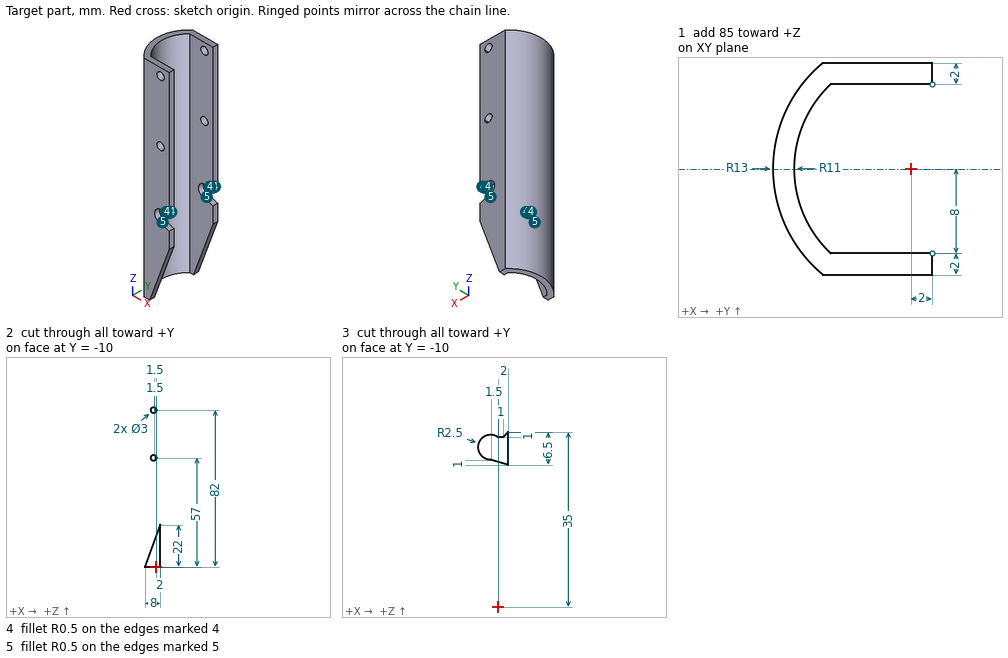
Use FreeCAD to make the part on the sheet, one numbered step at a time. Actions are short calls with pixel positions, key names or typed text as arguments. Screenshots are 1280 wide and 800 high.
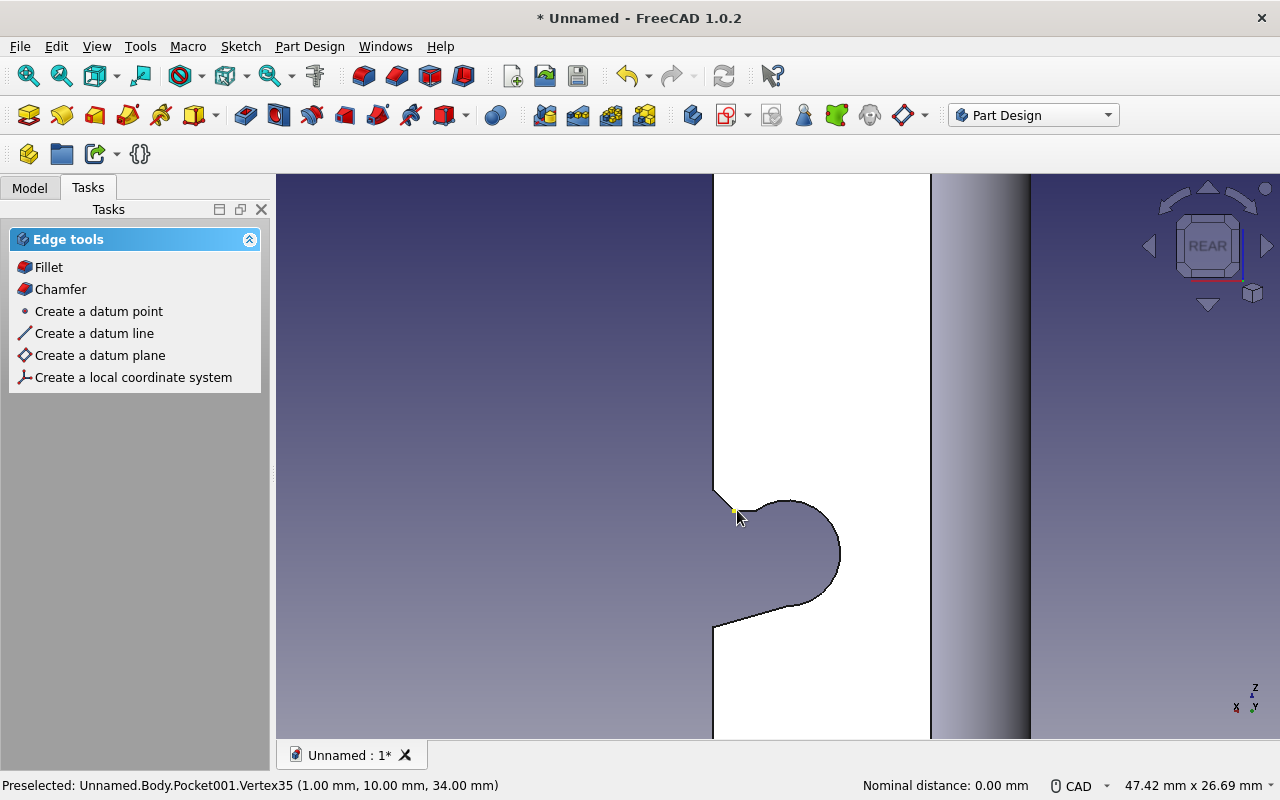
click(29, 76)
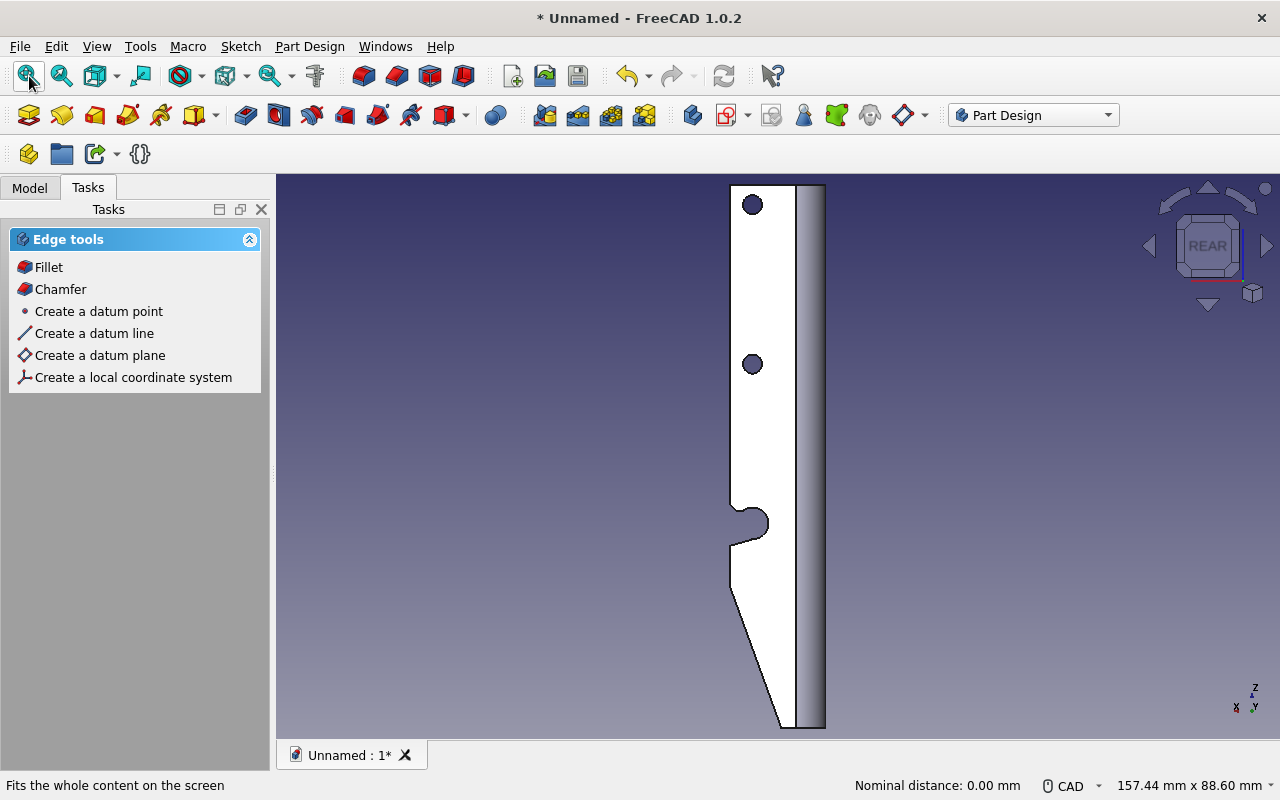
key(6)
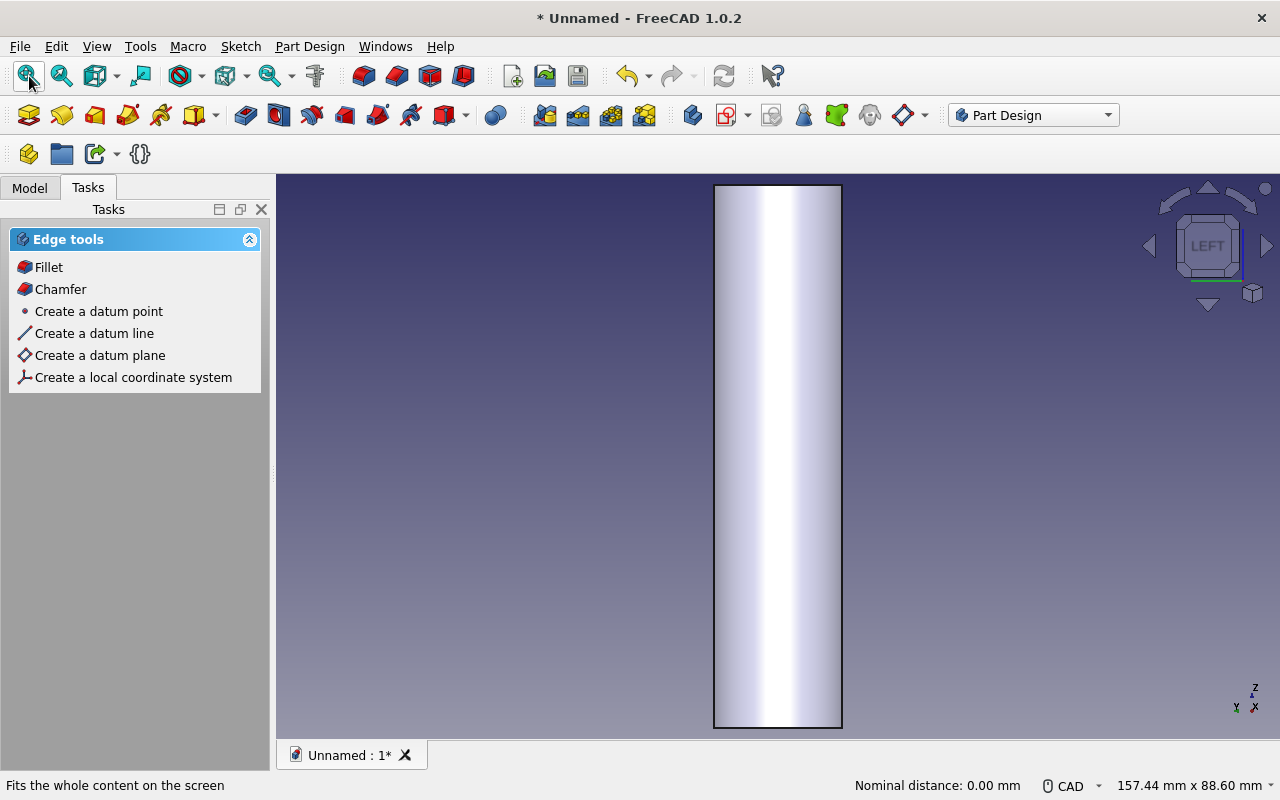
scroll(835, 510, up, 6)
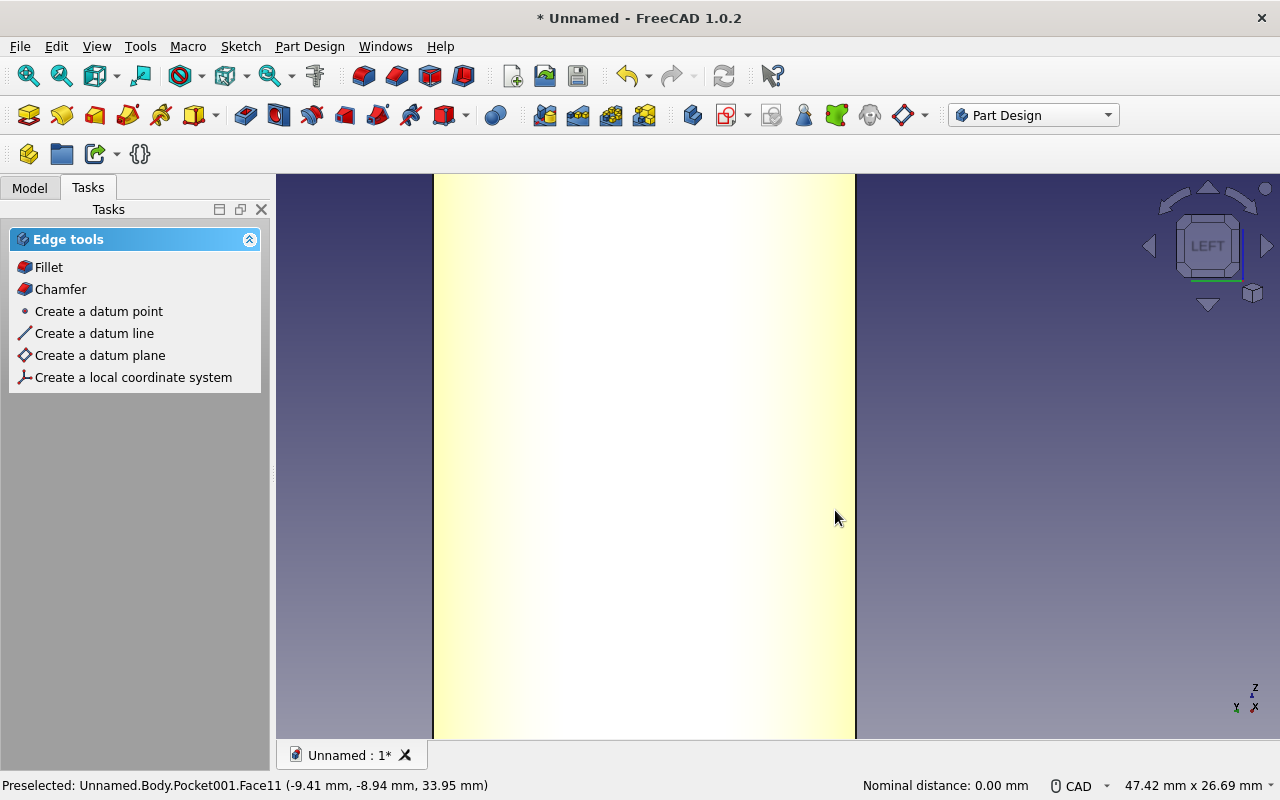
key(v)
key(f)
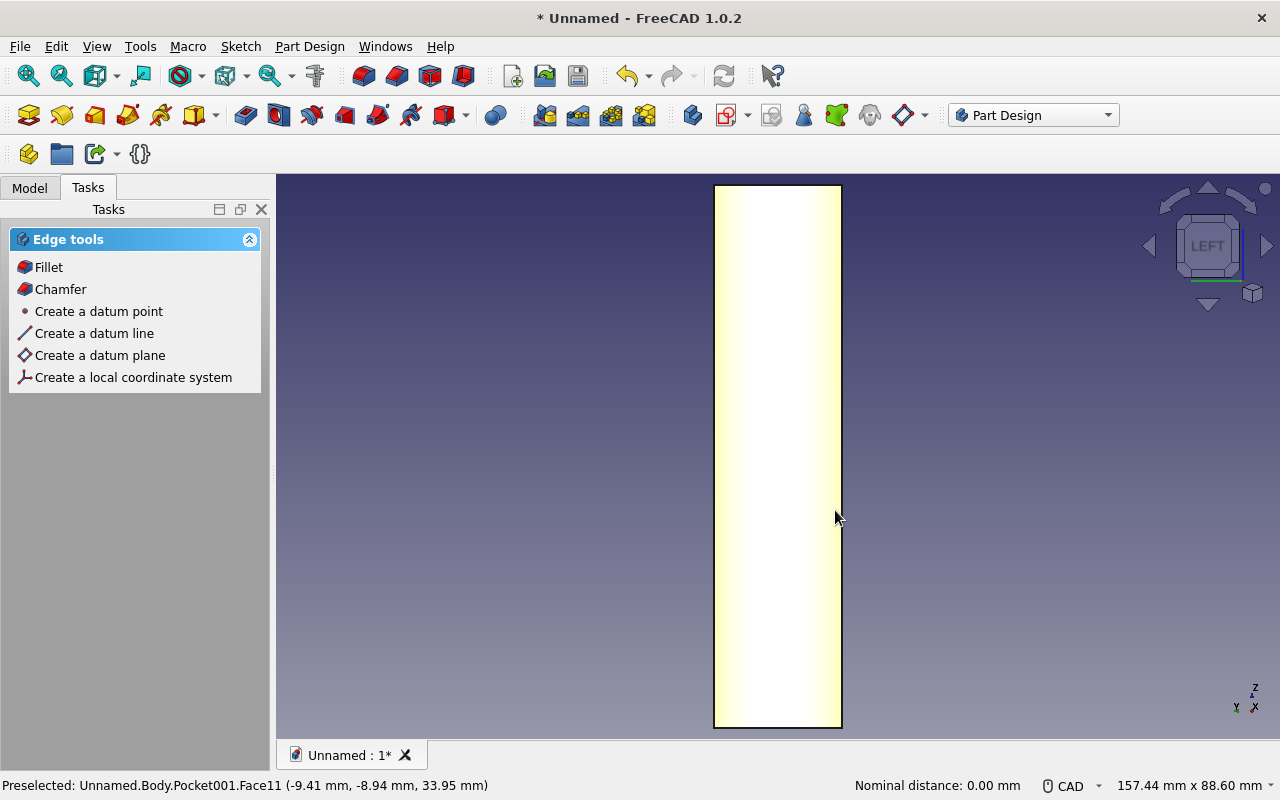
key(v)
key(3)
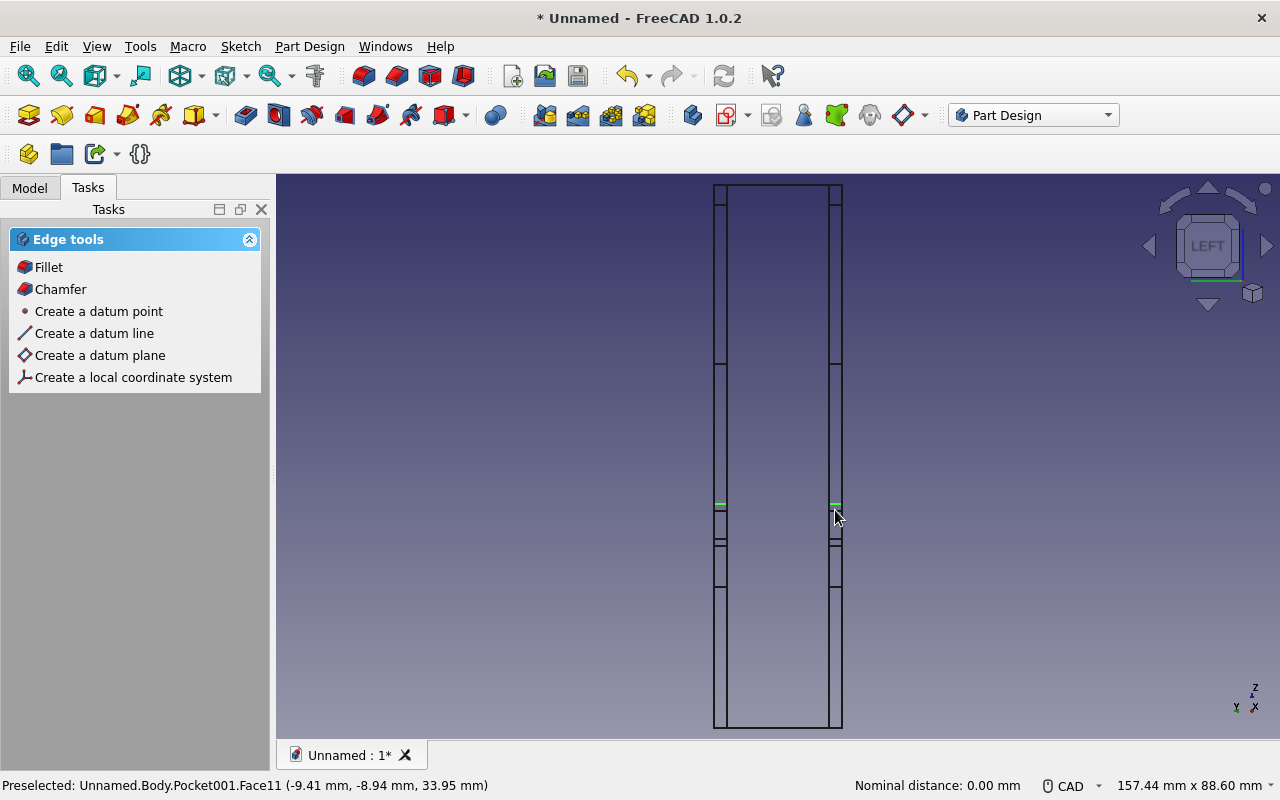
key(0)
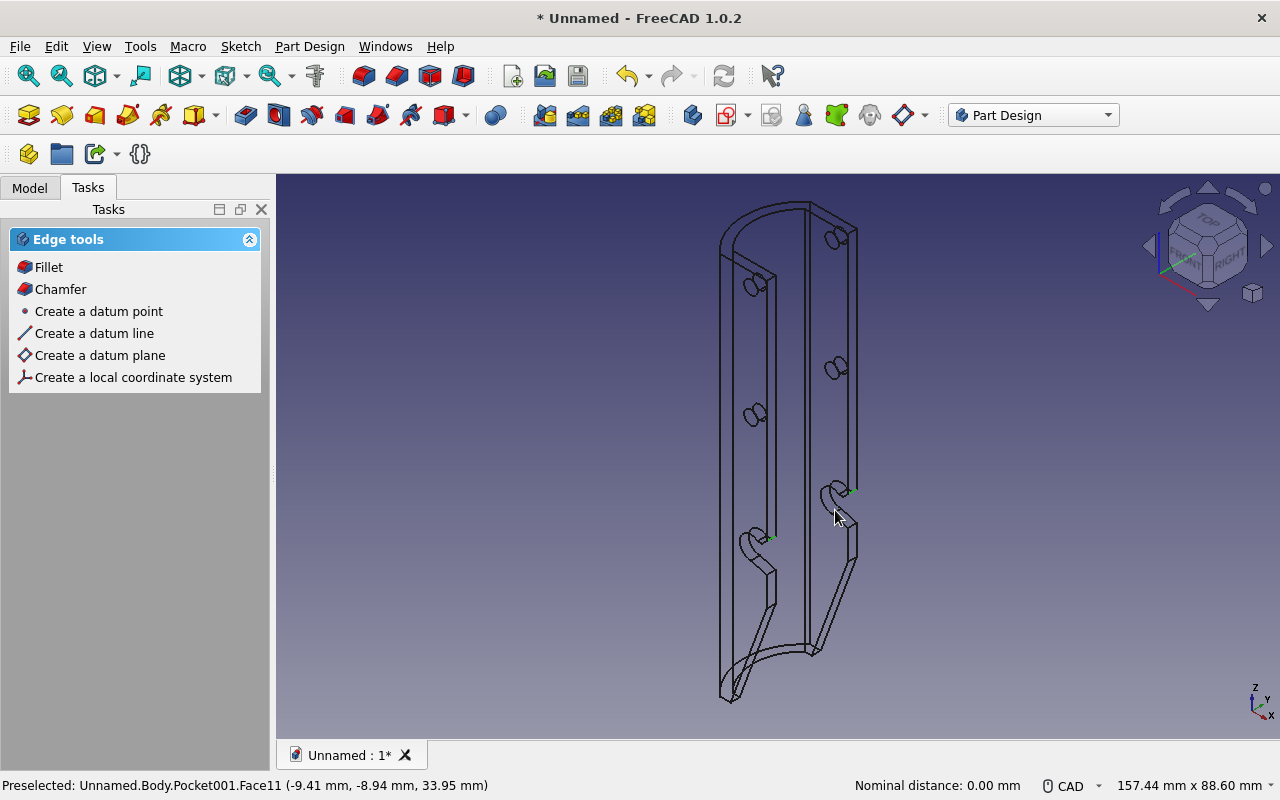
scroll(767, 540, up, 6)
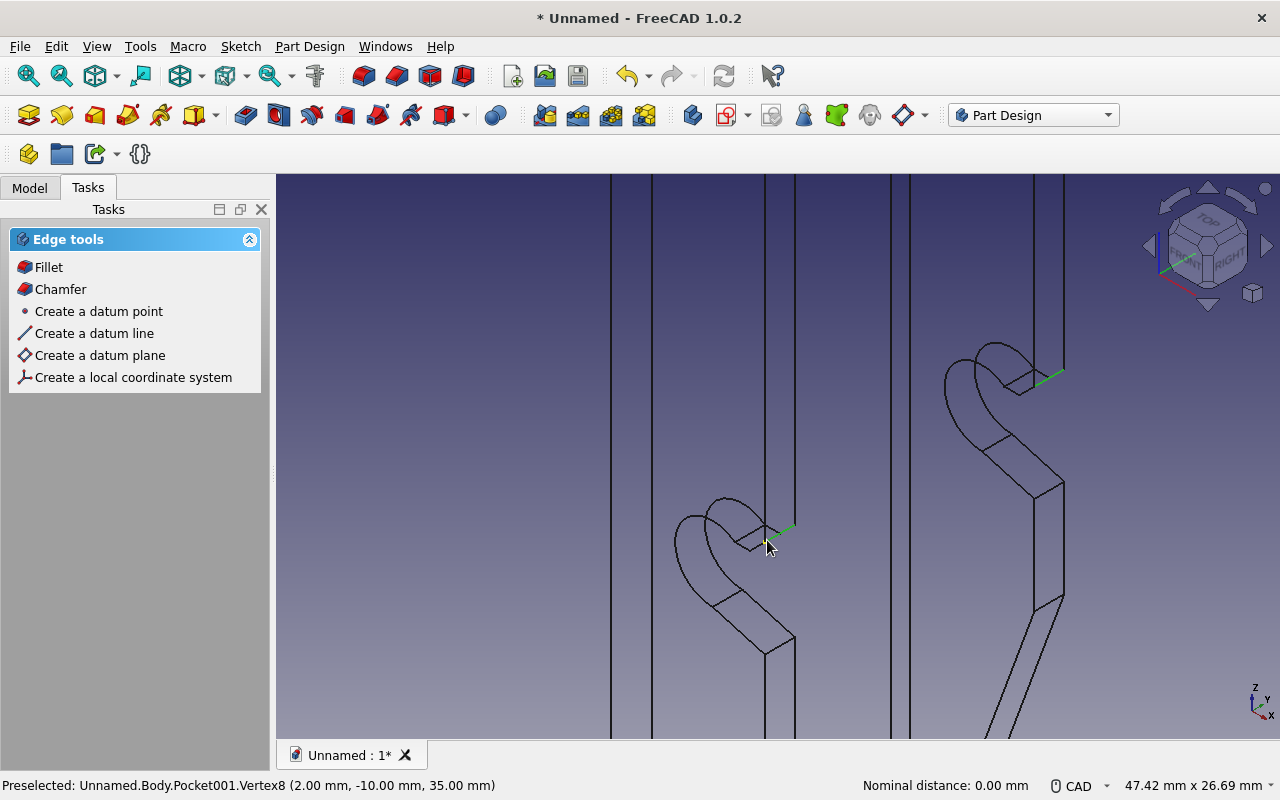
click(750, 533, ctrl)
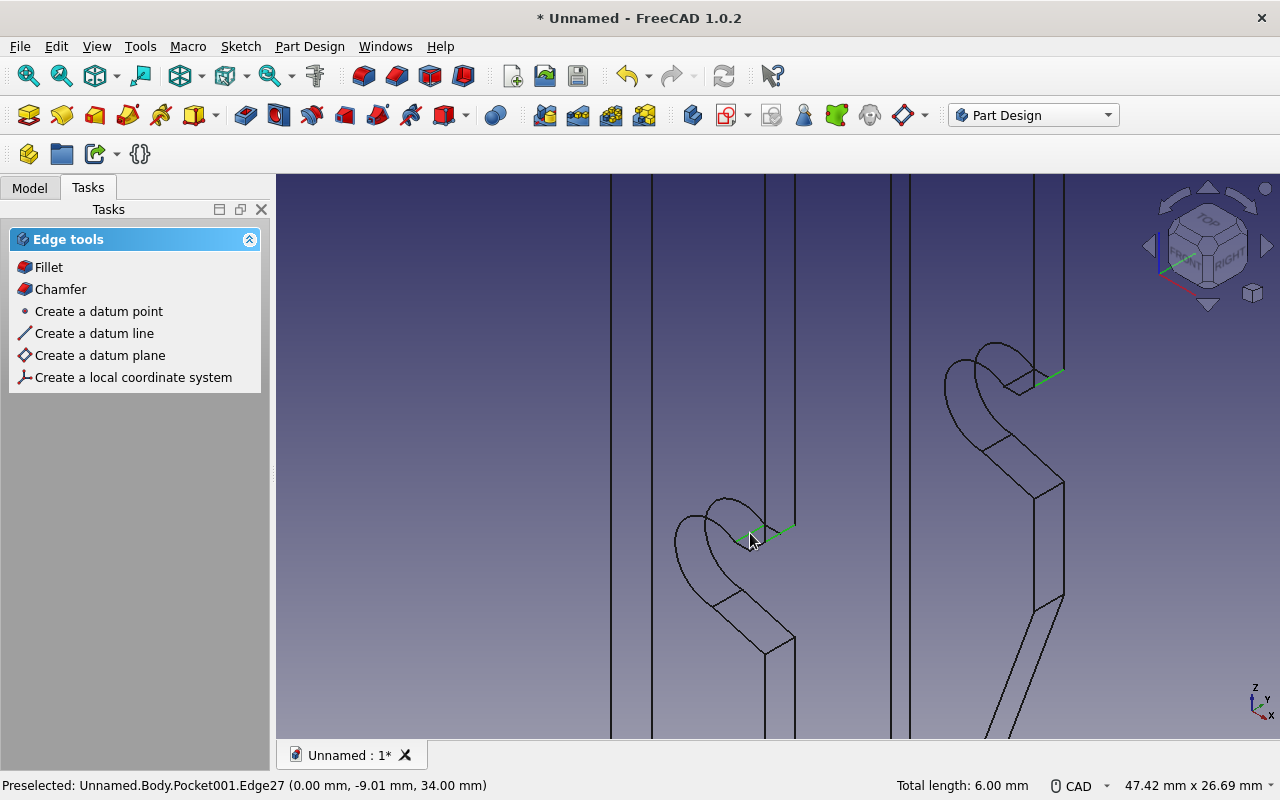
click(1019, 377, ctrl)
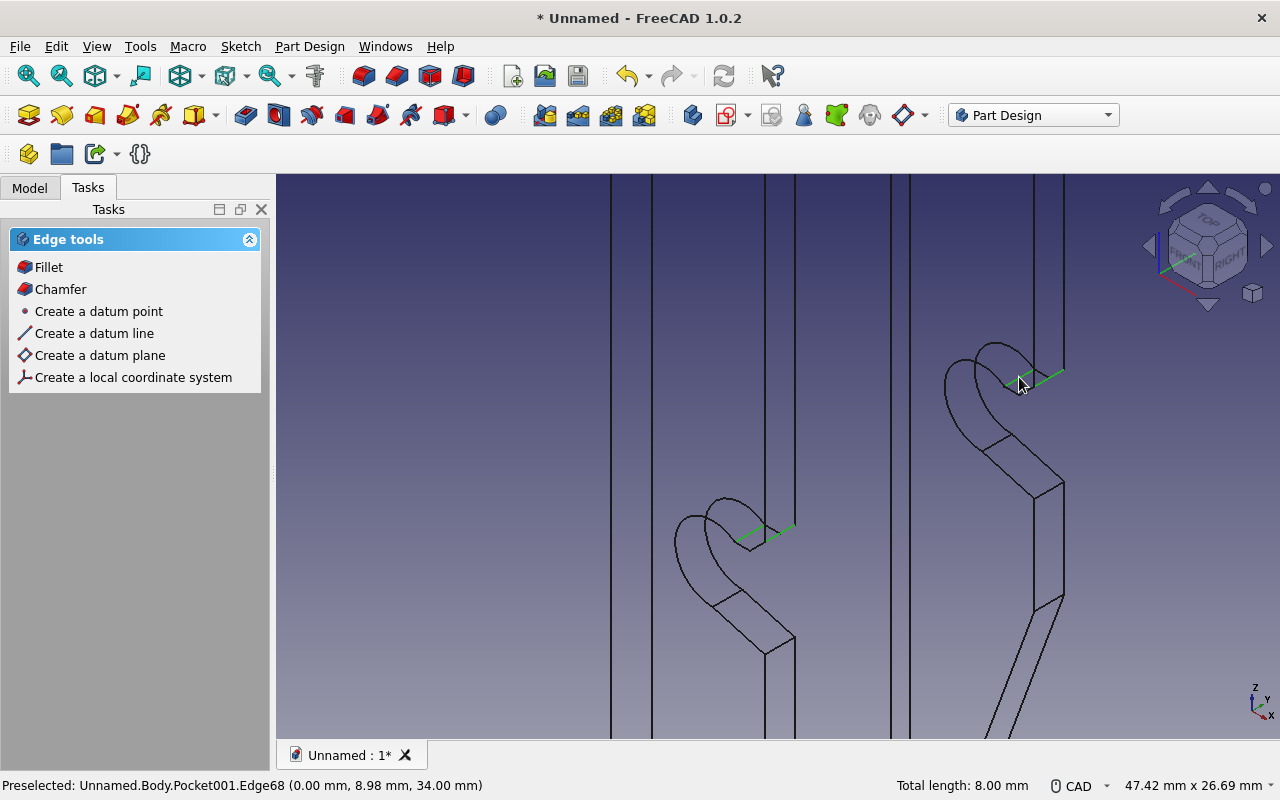
click(29, 76)